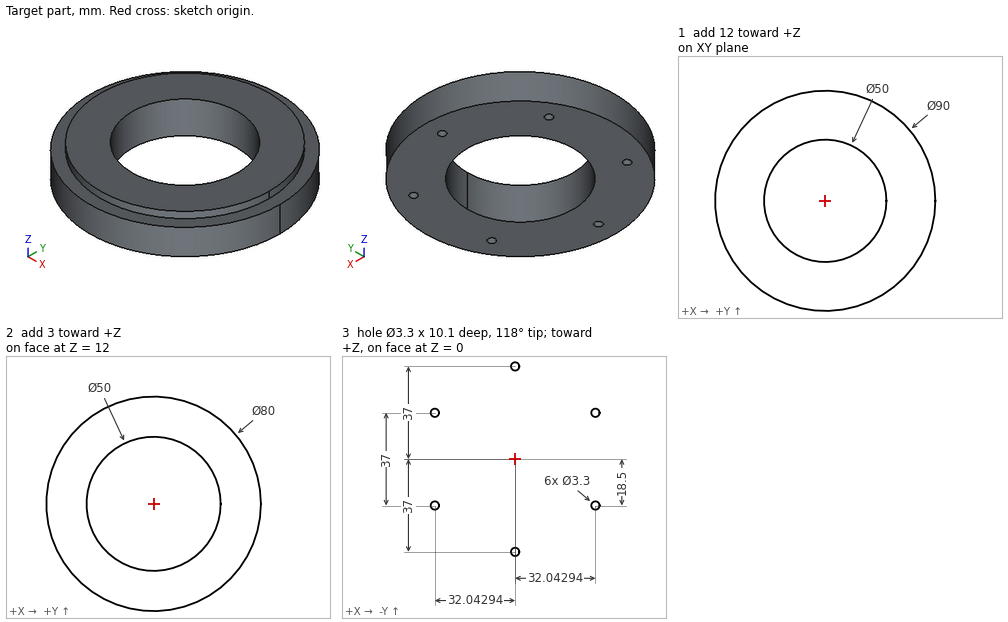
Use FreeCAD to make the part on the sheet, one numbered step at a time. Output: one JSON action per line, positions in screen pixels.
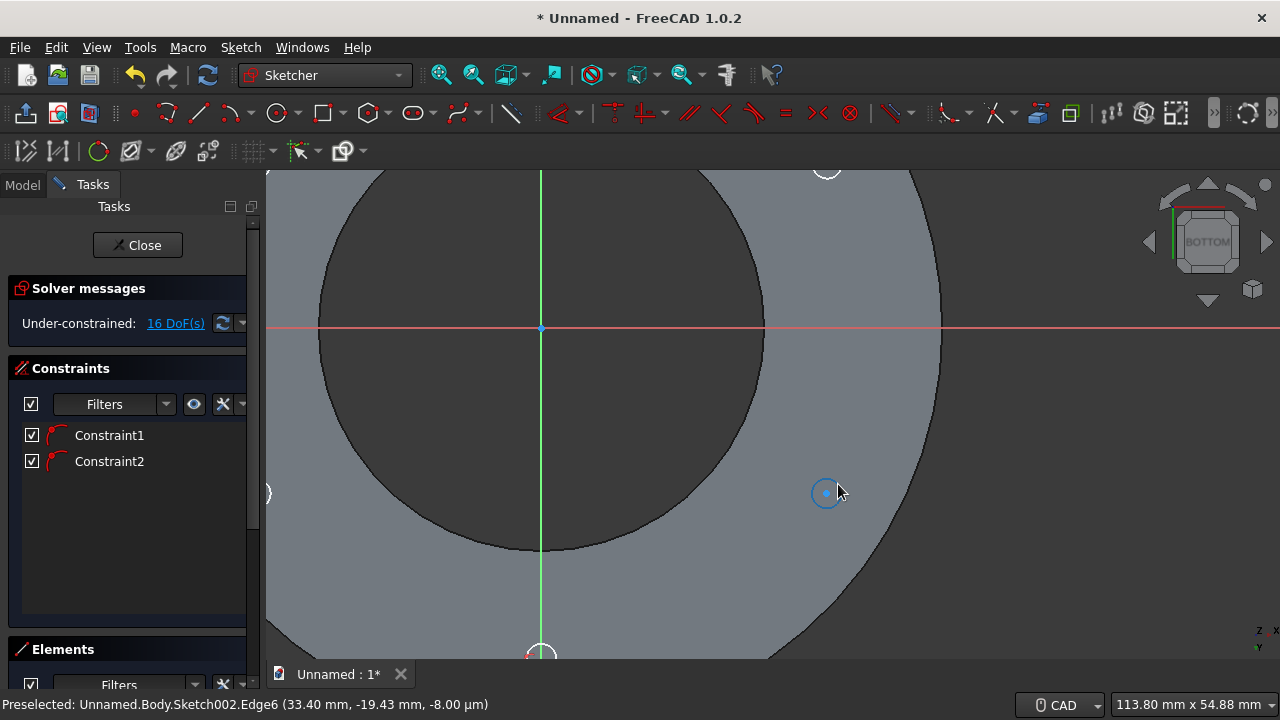
{"action": "left_click", "coordinate": [837, 483]}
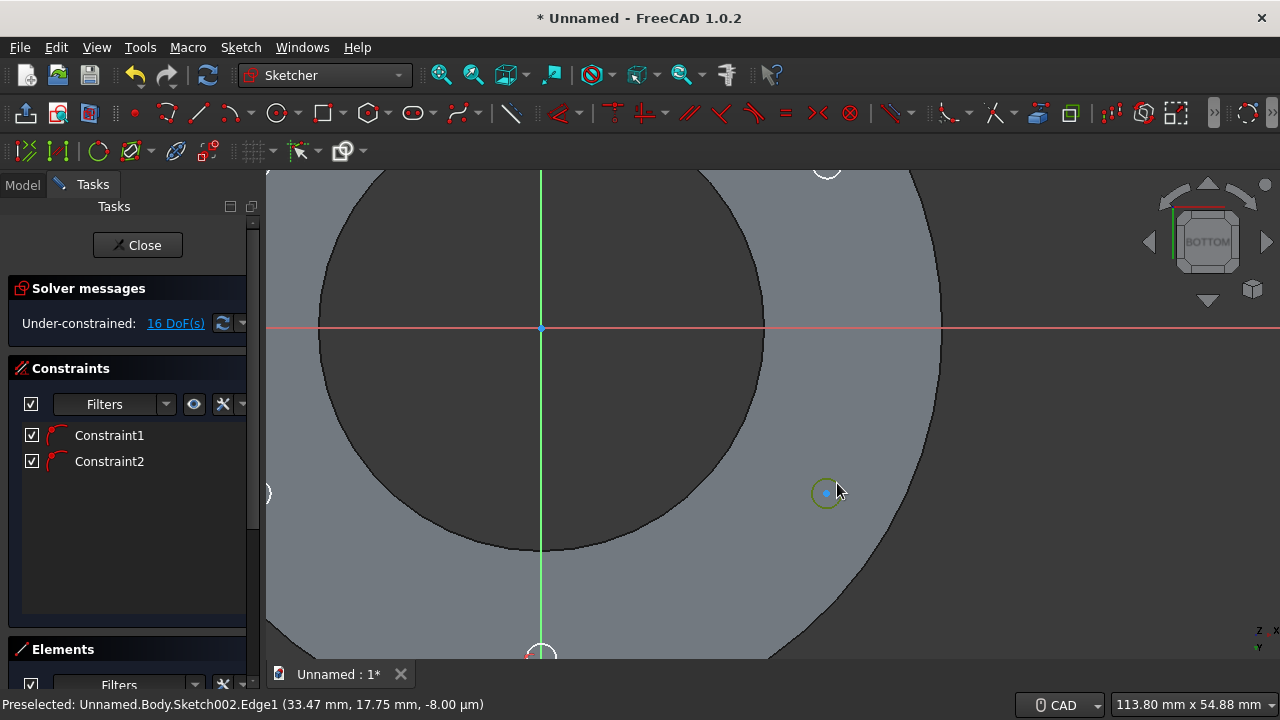
{"action": "scroll", "coordinate": [838, 485], "scroll_direction": "down", "scroll_amount": 4}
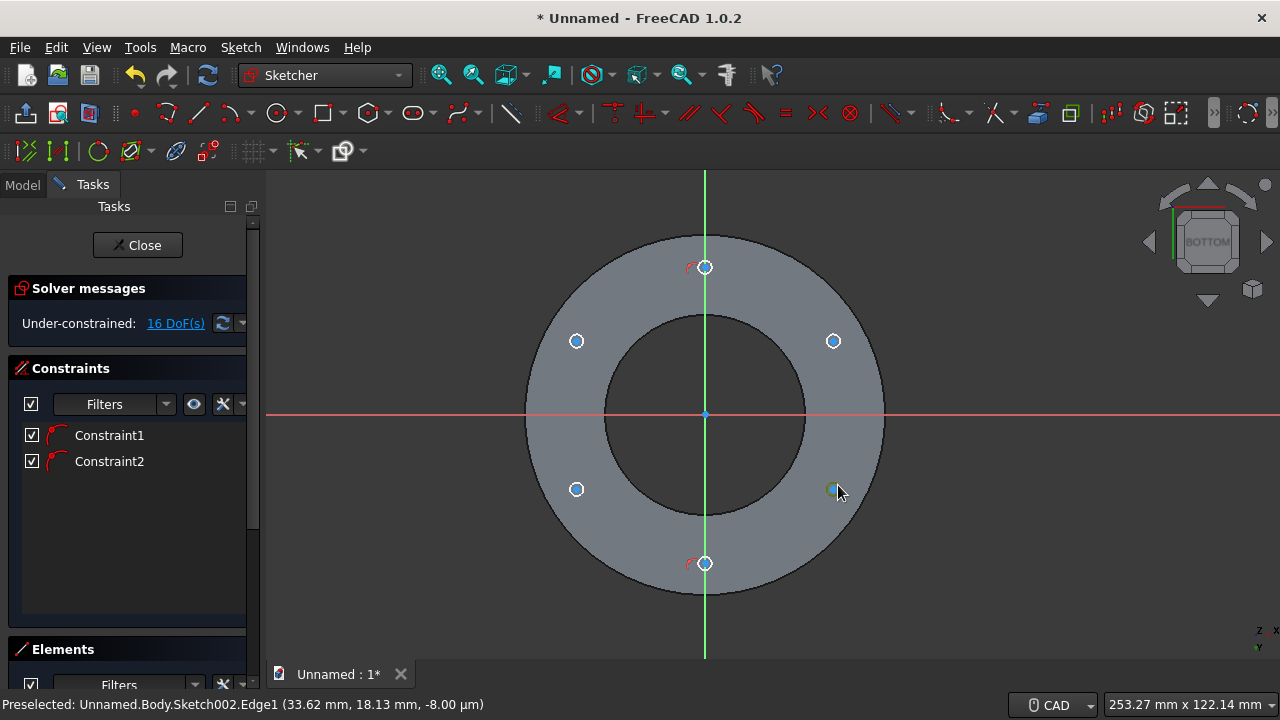
{"action": "scroll", "coordinate": [710, 559], "scroll_direction": "up", "scroll_amount": 6}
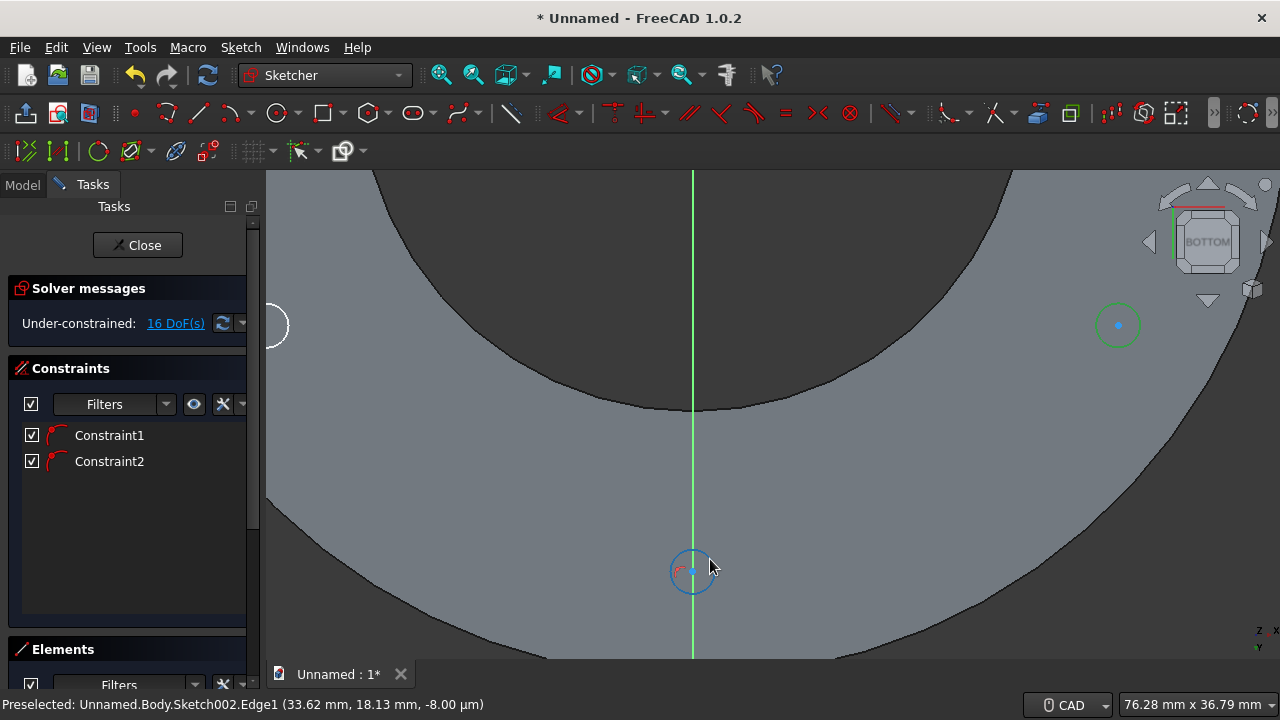
{"action": "left_click", "coordinate": [708, 556]}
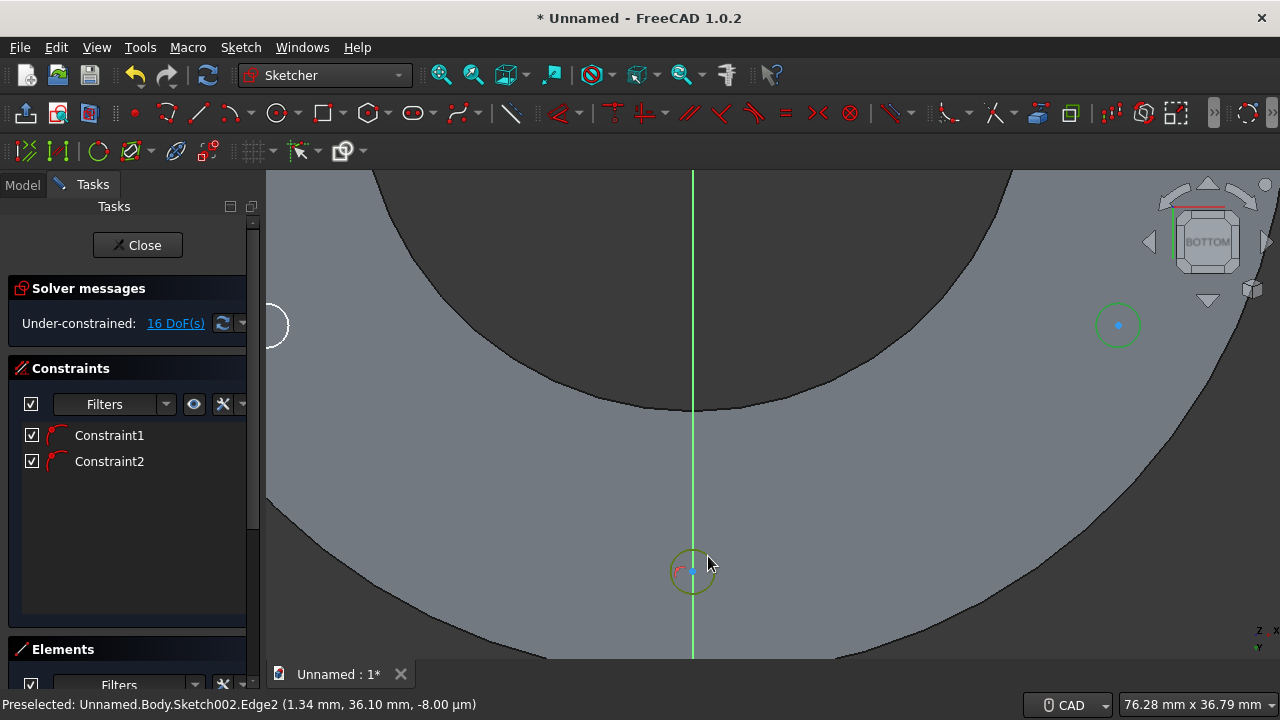
{"action": "scroll", "coordinate": [710, 559], "scroll_direction": "down", "scroll_amount": 6}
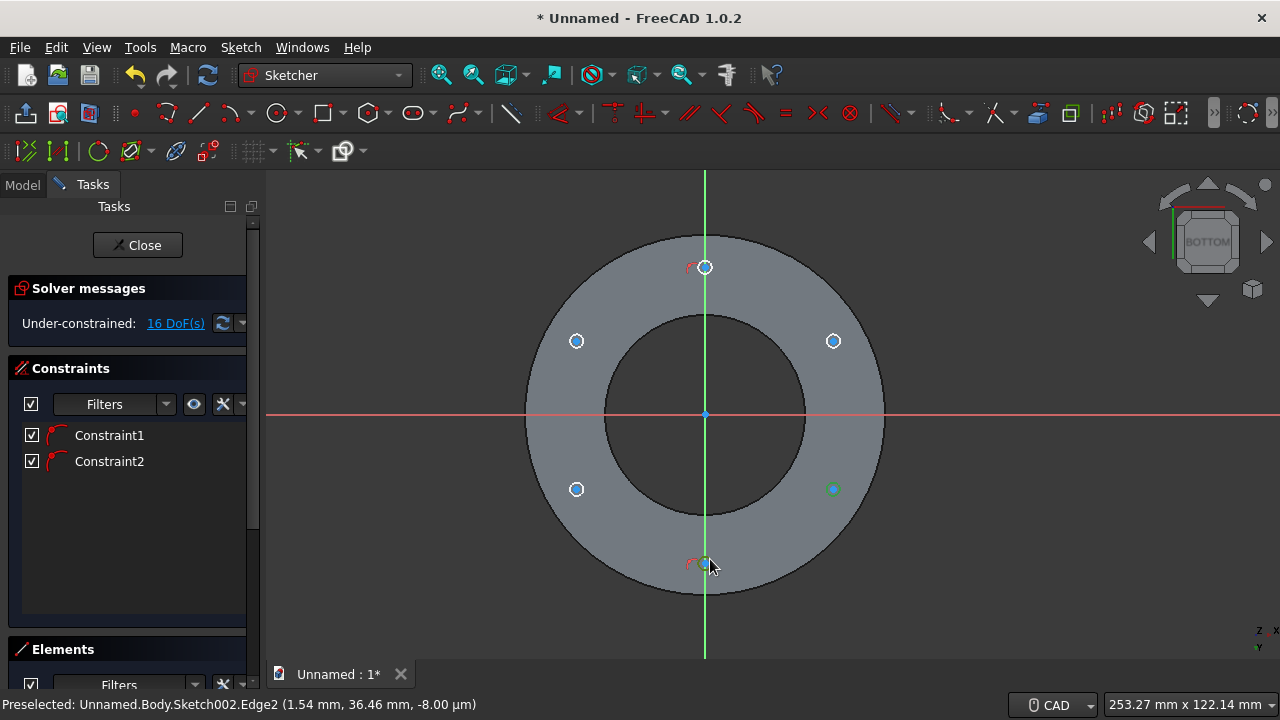
{"action": "scroll", "coordinate": [581, 485], "scroll_direction": "up", "scroll_amount": 4}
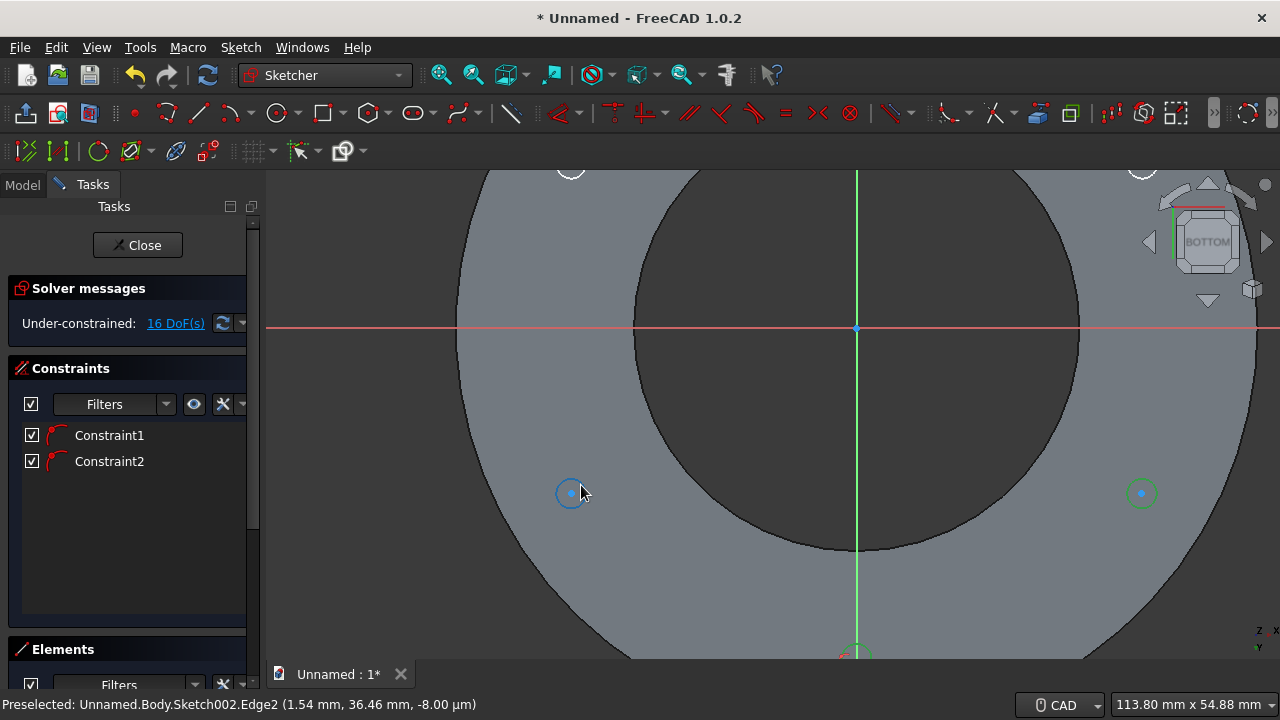
{"action": "left_click", "coordinate": [582, 483]}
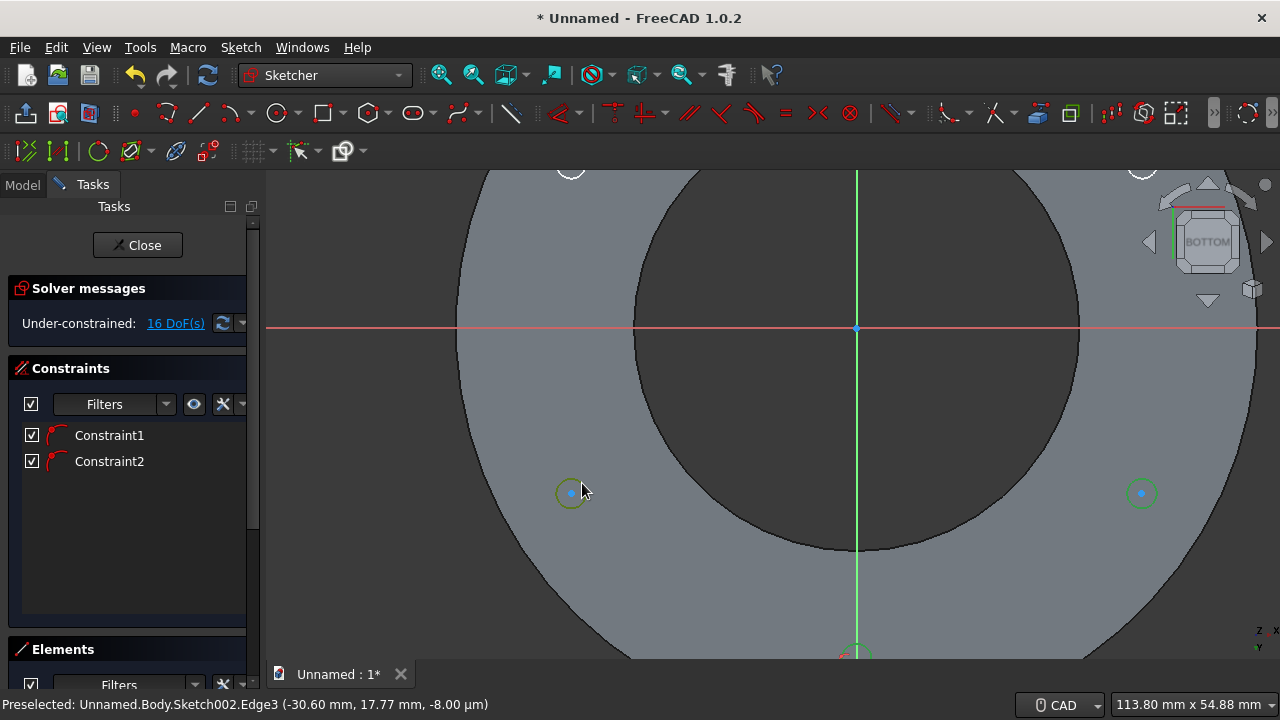
{"action": "scroll", "coordinate": [580, 485], "scroll_direction": "down", "scroll_amount": 4}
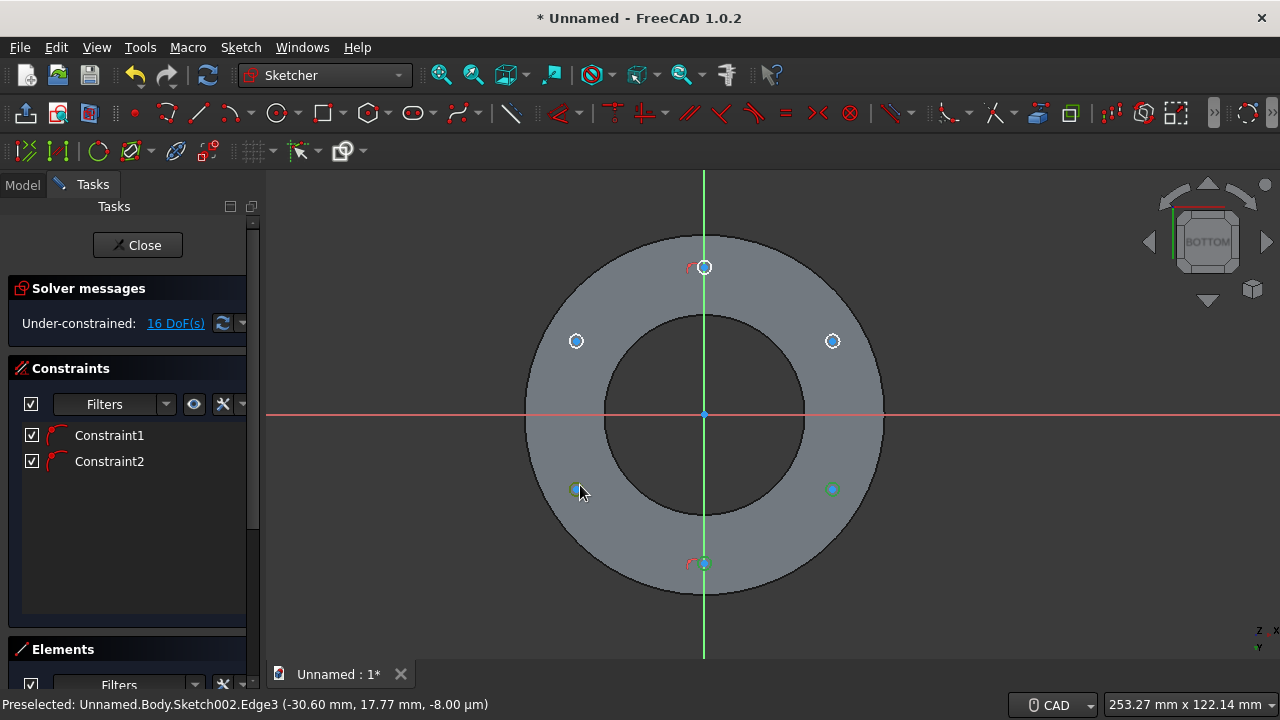
{"action": "scroll", "coordinate": [581, 336], "scroll_direction": "up", "scroll_amount": 4}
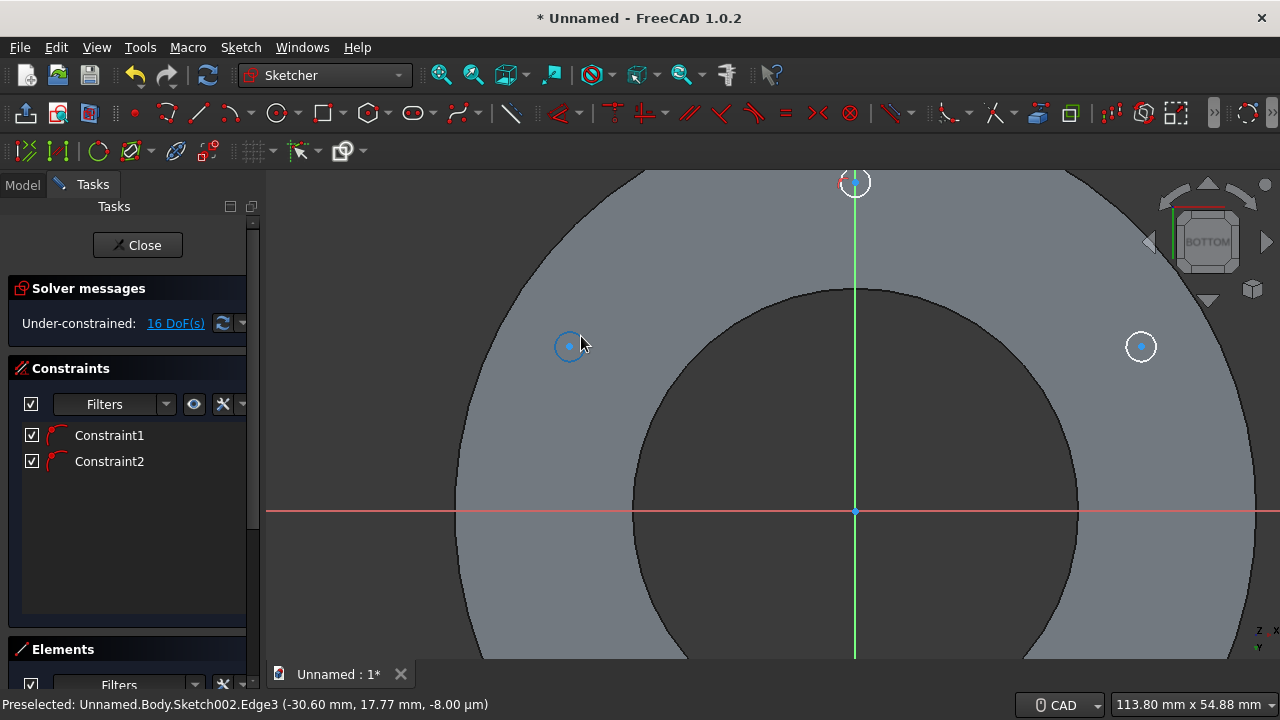
{"action": "left_click", "coordinate": [580, 336]}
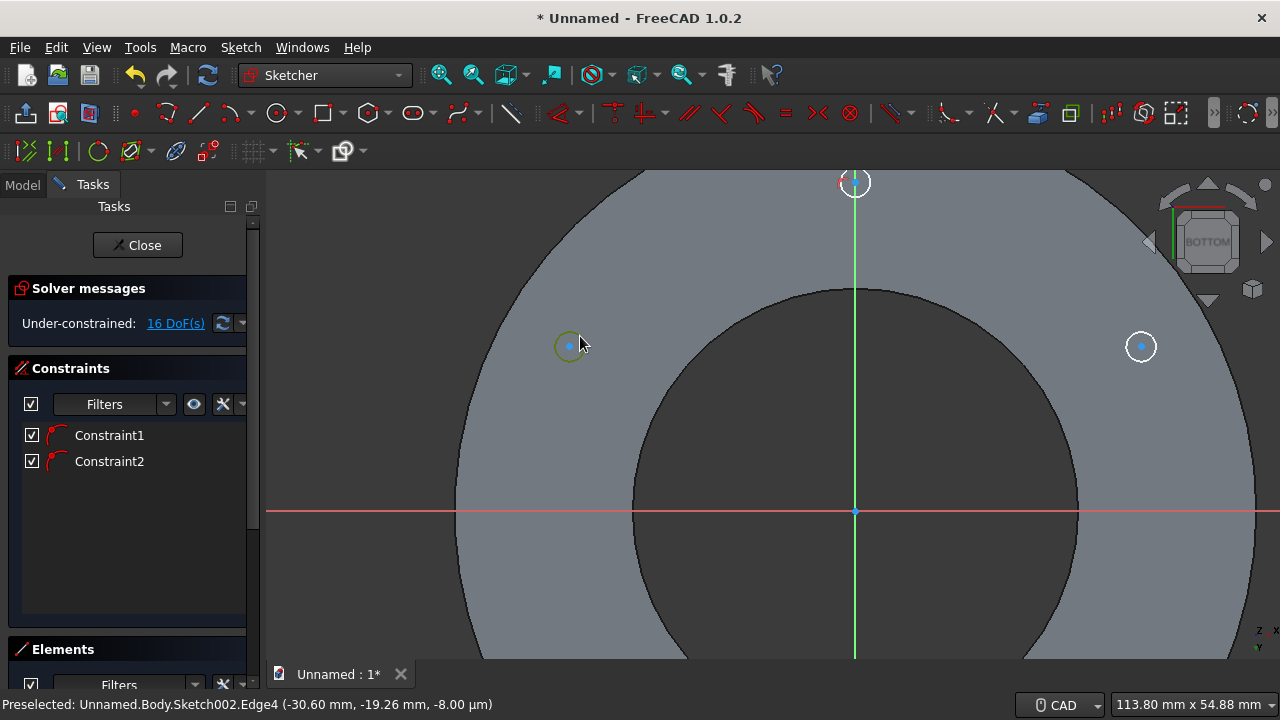
{"action": "scroll", "coordinate": [581, 335], "scroll_direction": "down", "scroll_amount": 4}